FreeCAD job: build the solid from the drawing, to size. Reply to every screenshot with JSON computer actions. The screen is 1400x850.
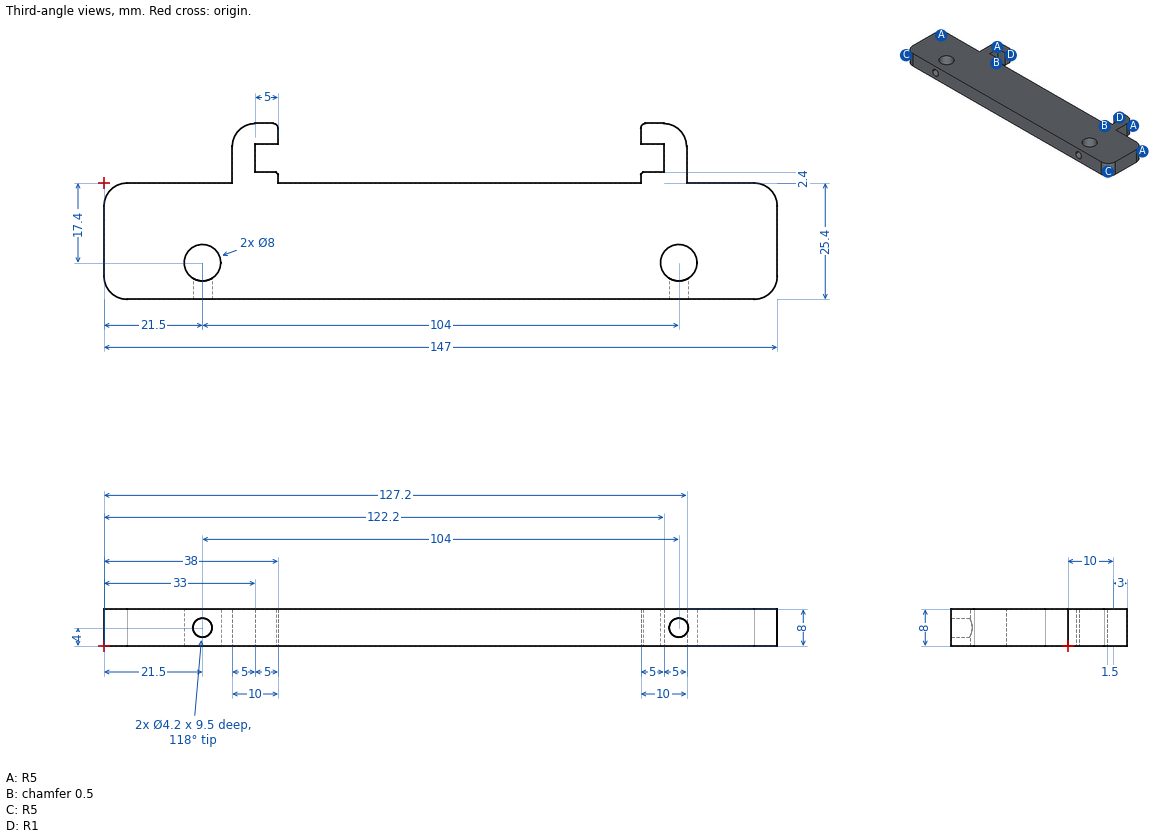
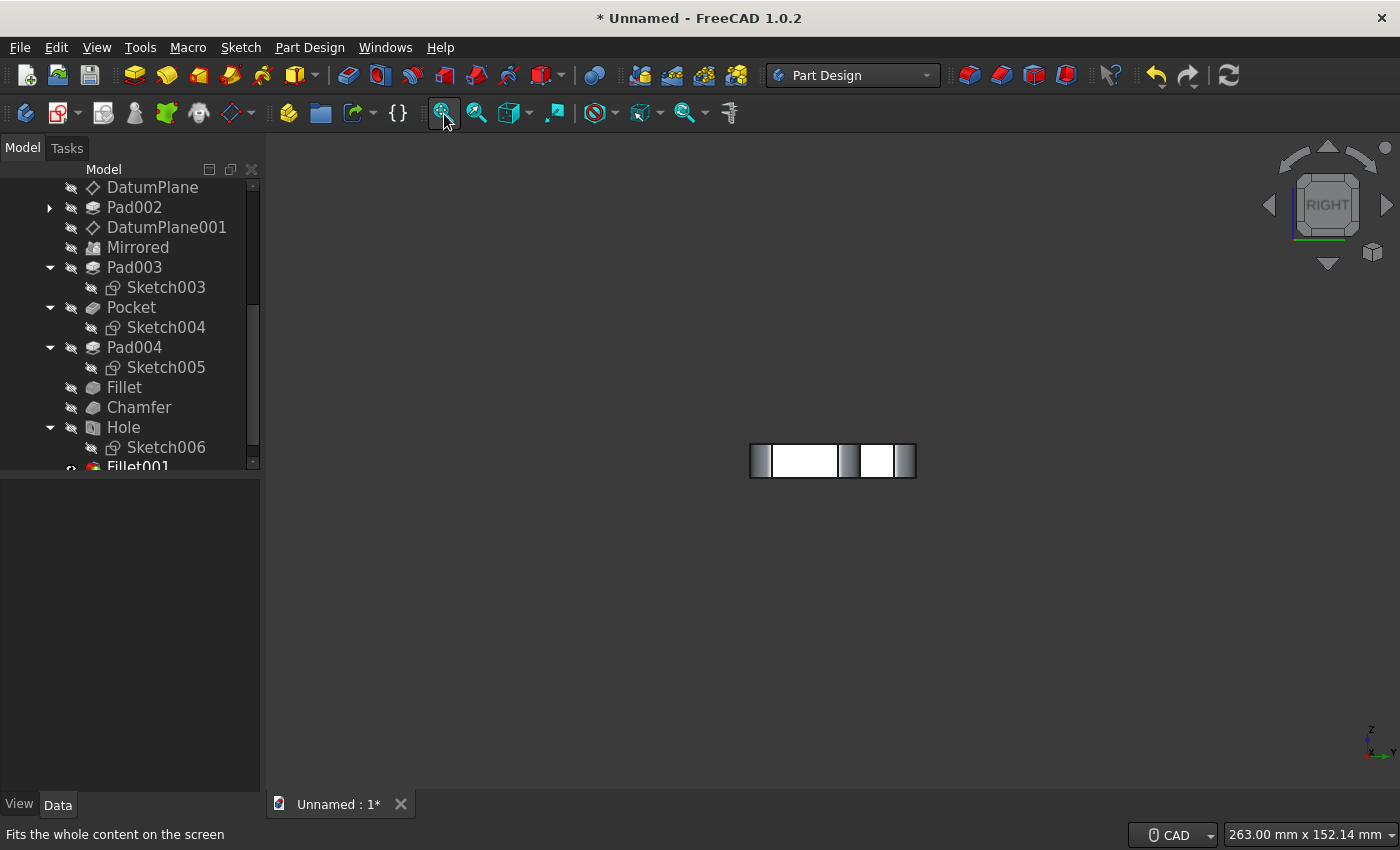
{"action": "key", "text": "5"}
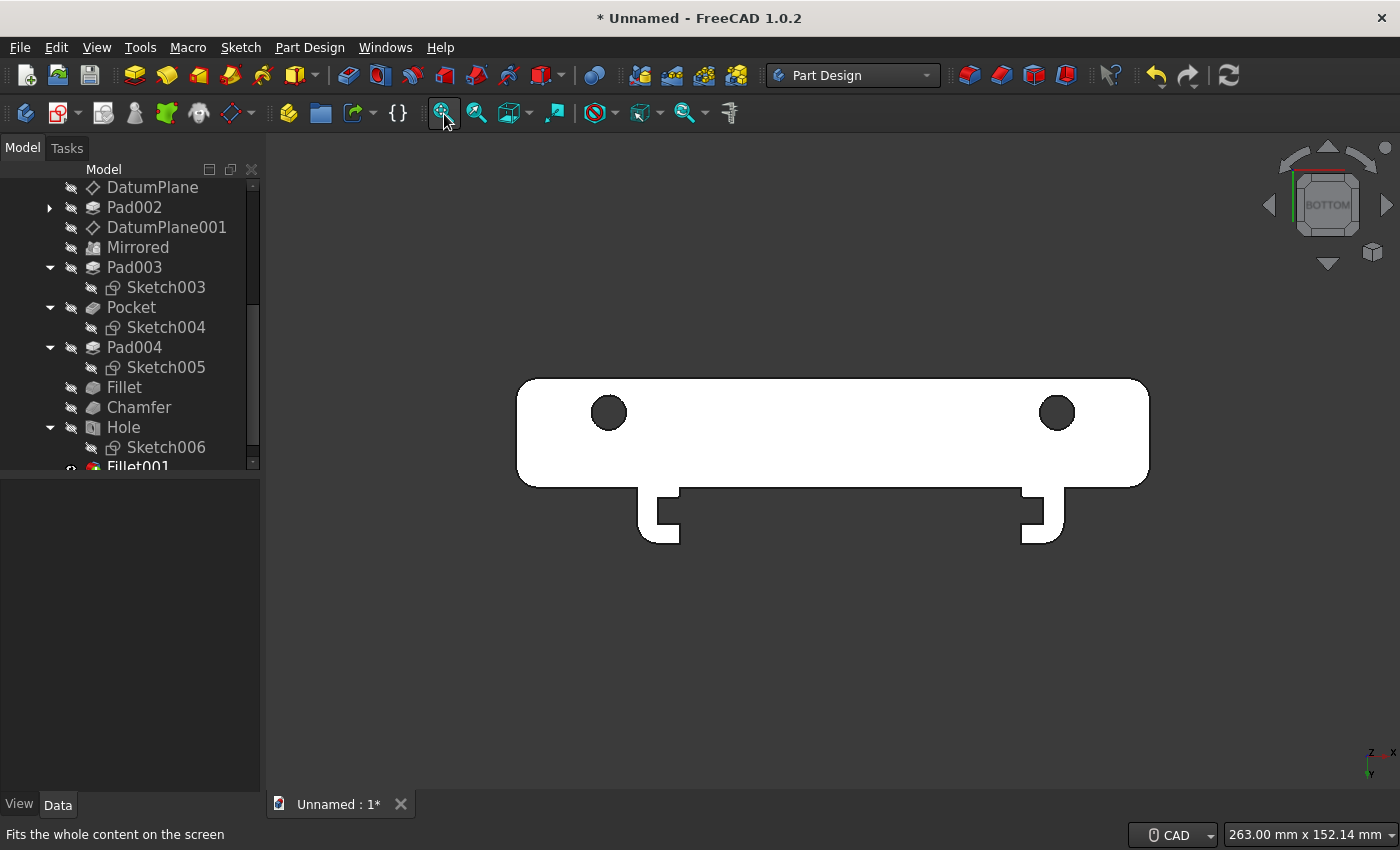
{"action": "key", "text": "4"}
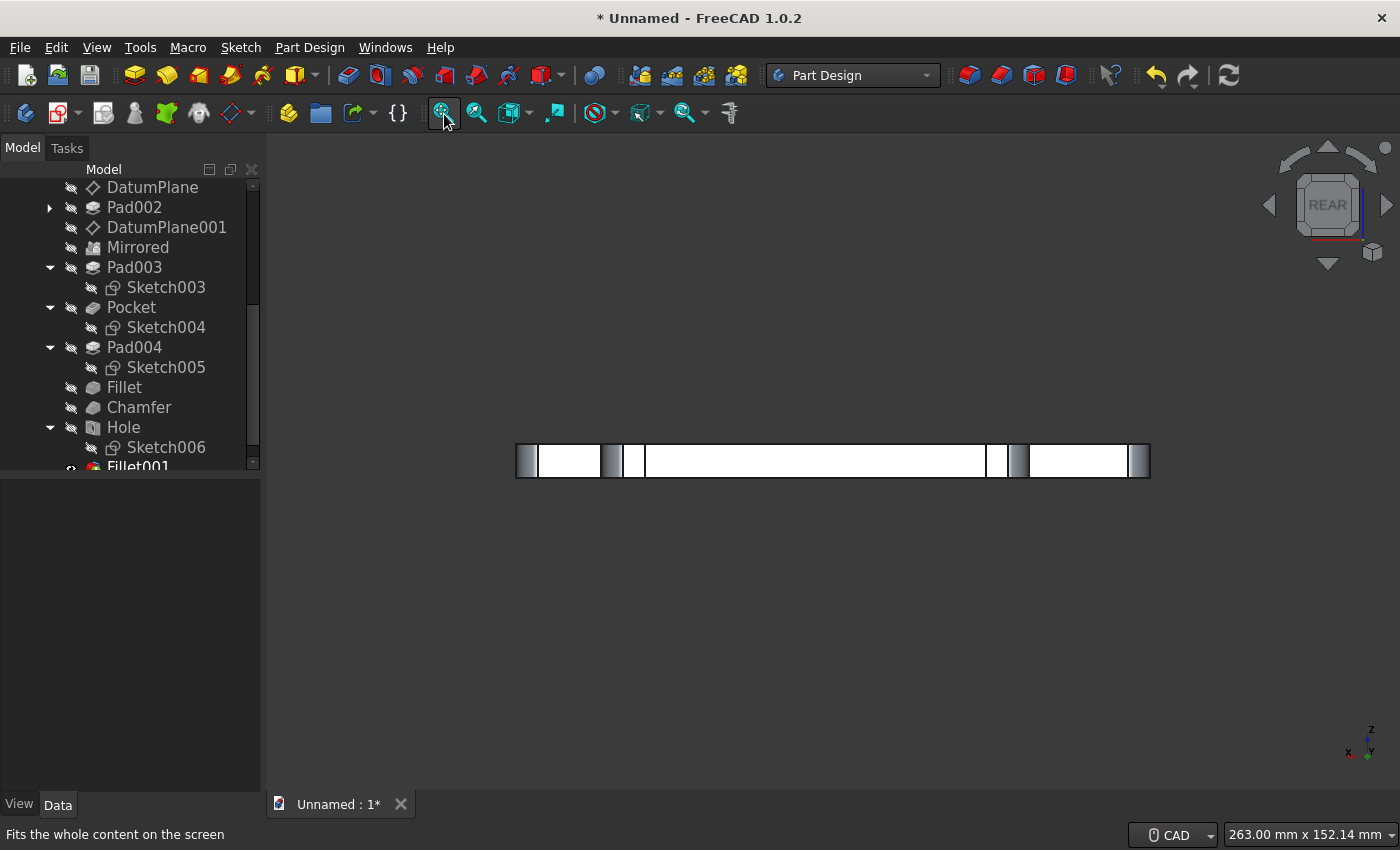
{"action": "left_click", "coordinate": [986, 460]}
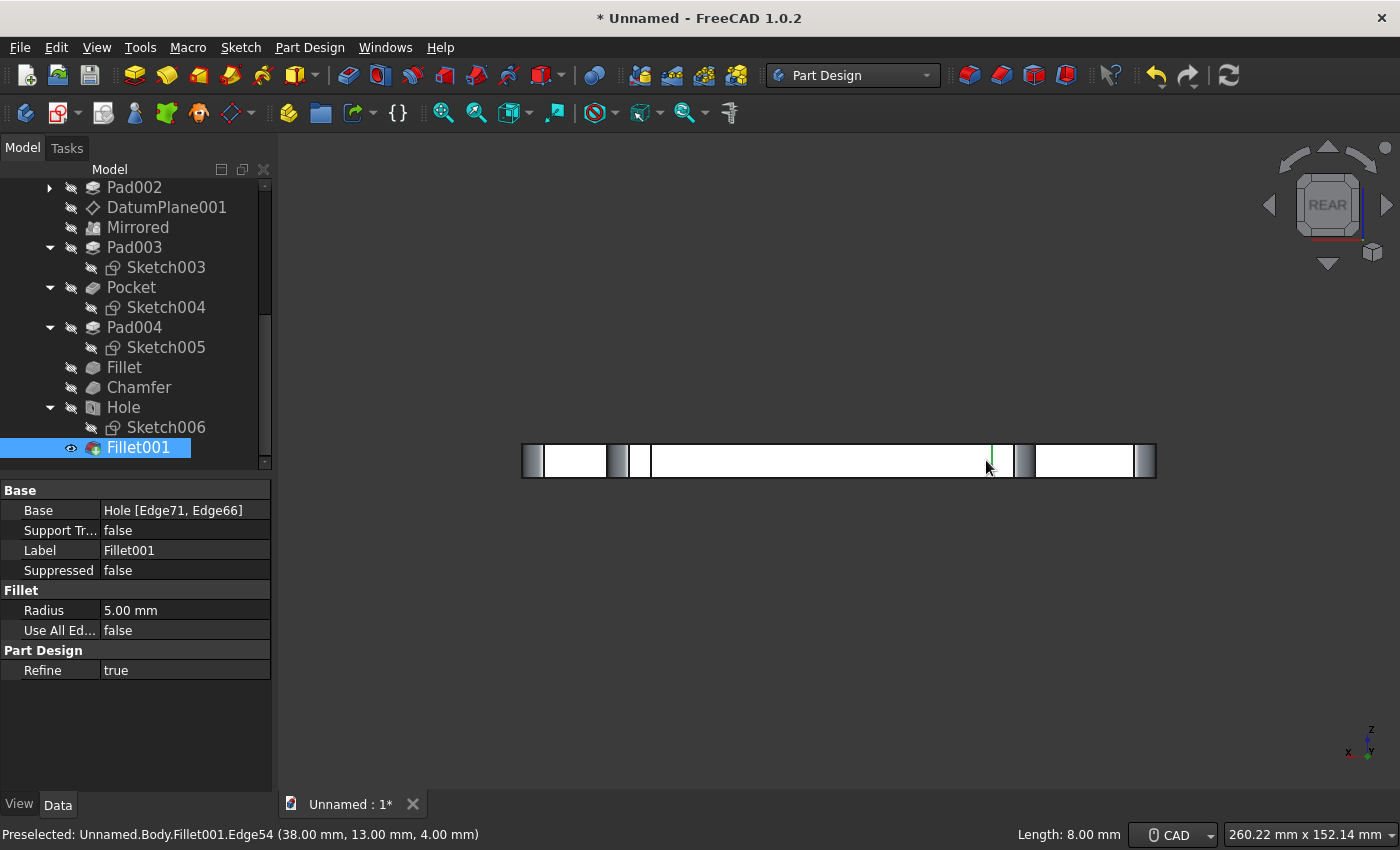
{"action": "left_click", "coordinate": [651, 460], "text": "ctrl"}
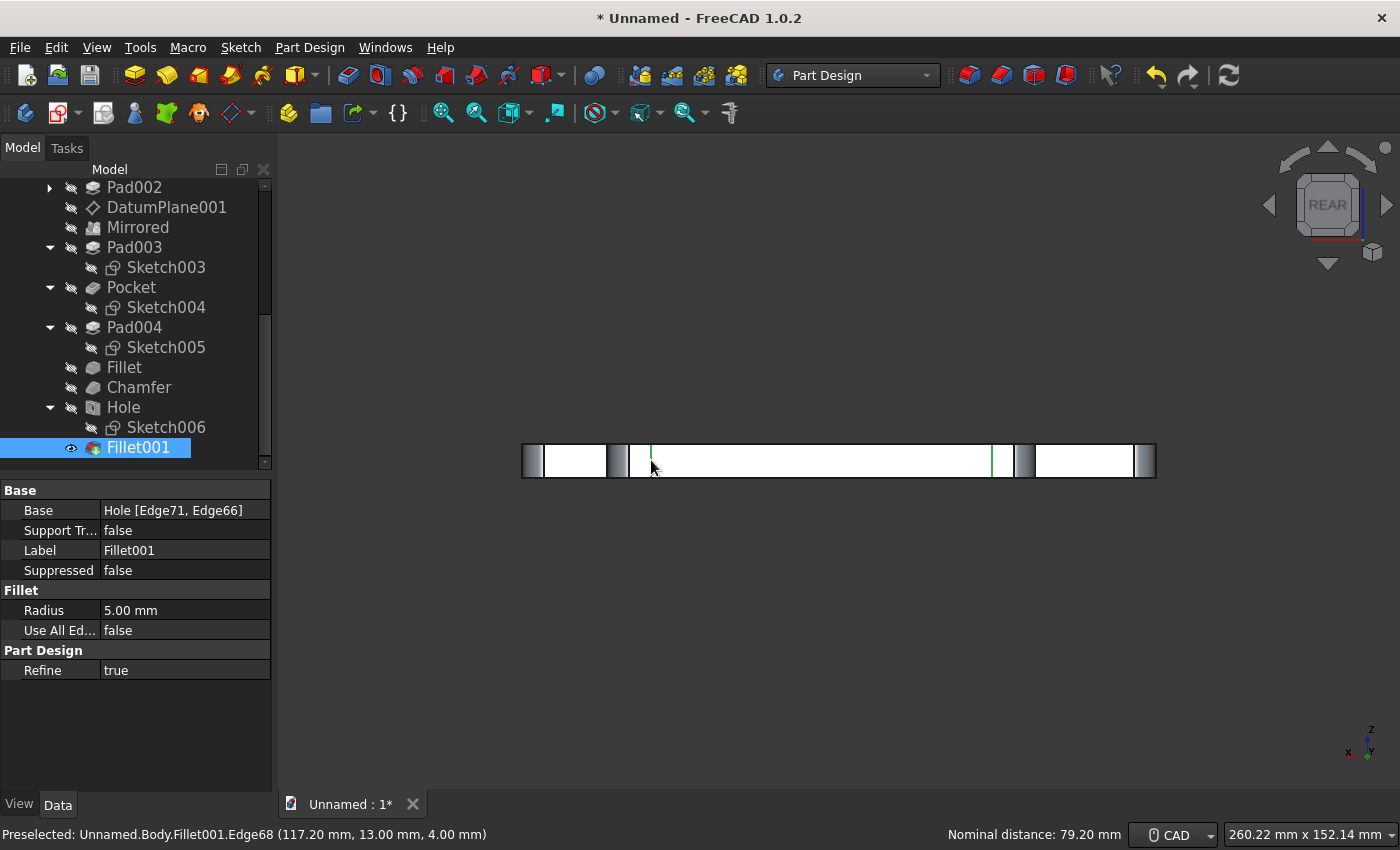
{"action": "left_click", "coordinate": [970, 76]}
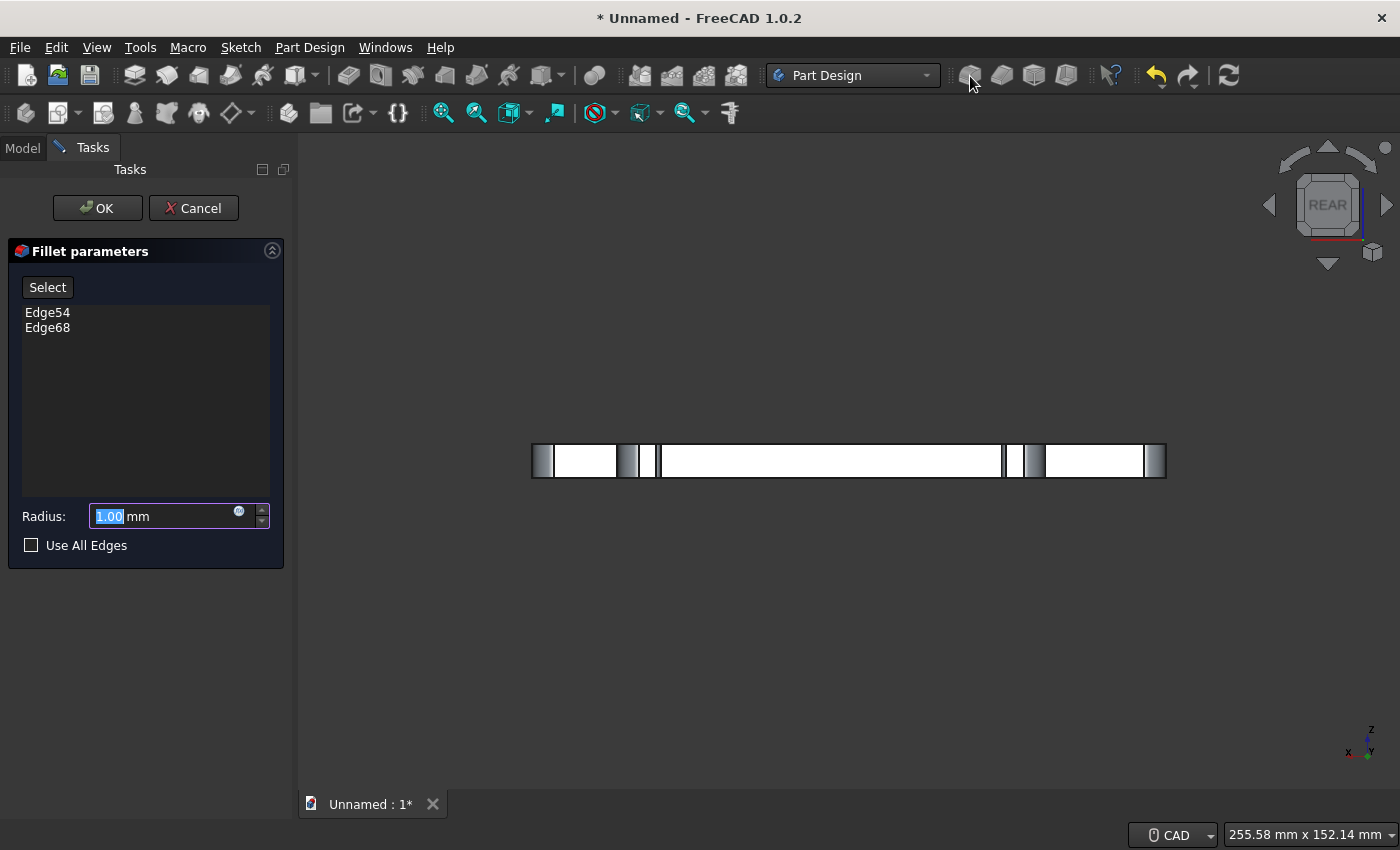
{"action": "type", "text": "1"}
{"action": "key", "text": "Tab"}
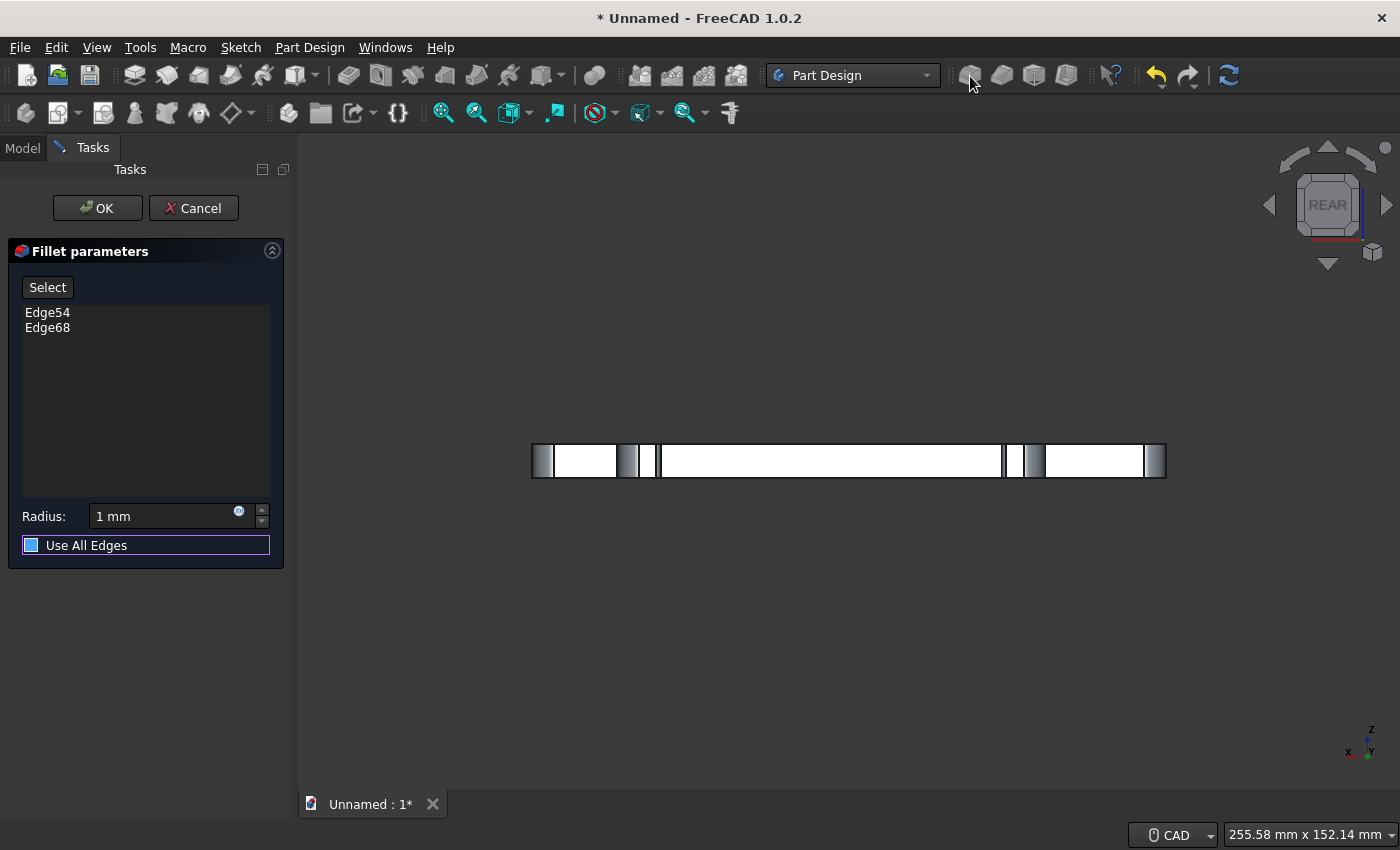
{"action": "left_click", "coordinate": [98, 208]}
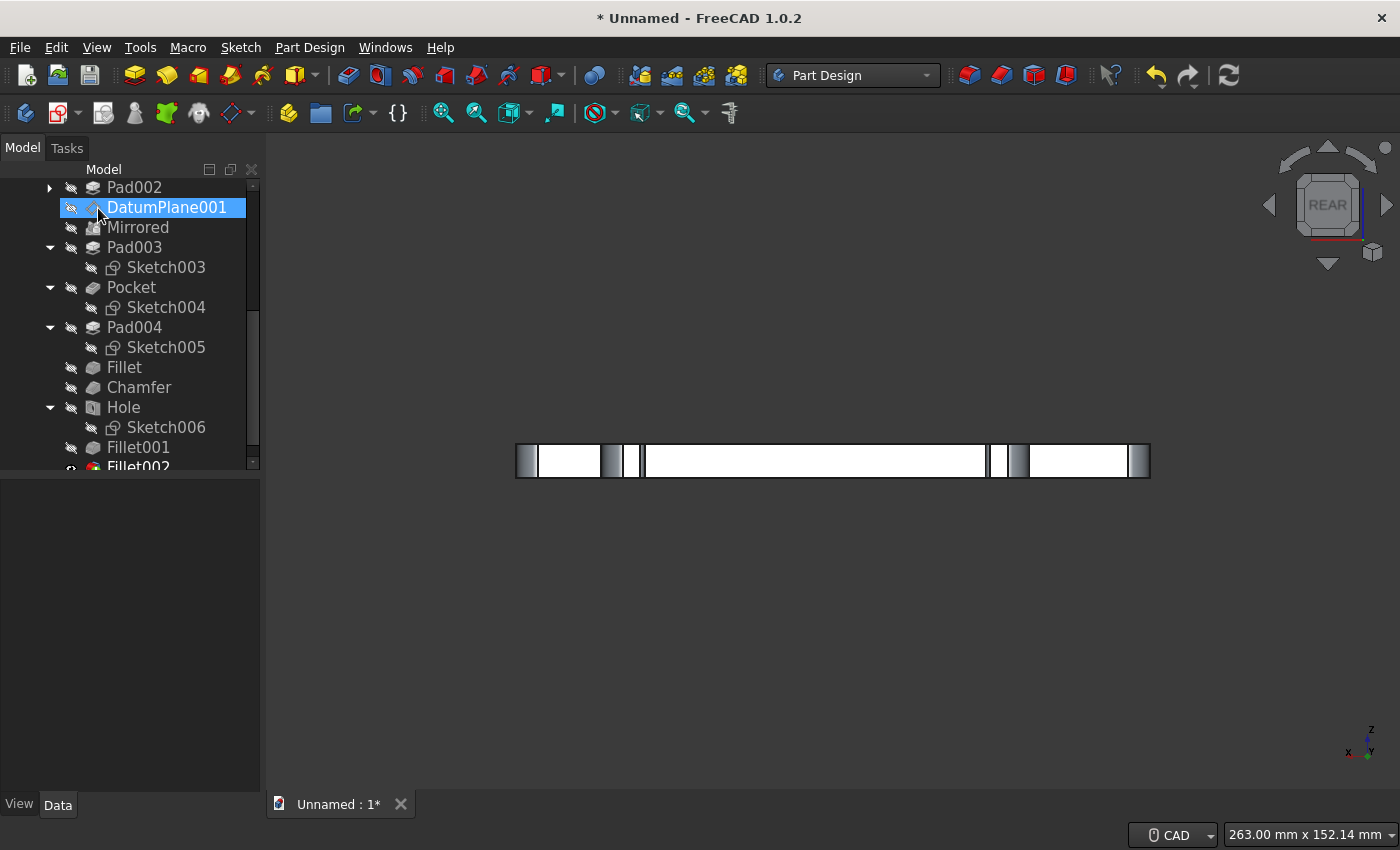
{"action": "key", "text": "0"}